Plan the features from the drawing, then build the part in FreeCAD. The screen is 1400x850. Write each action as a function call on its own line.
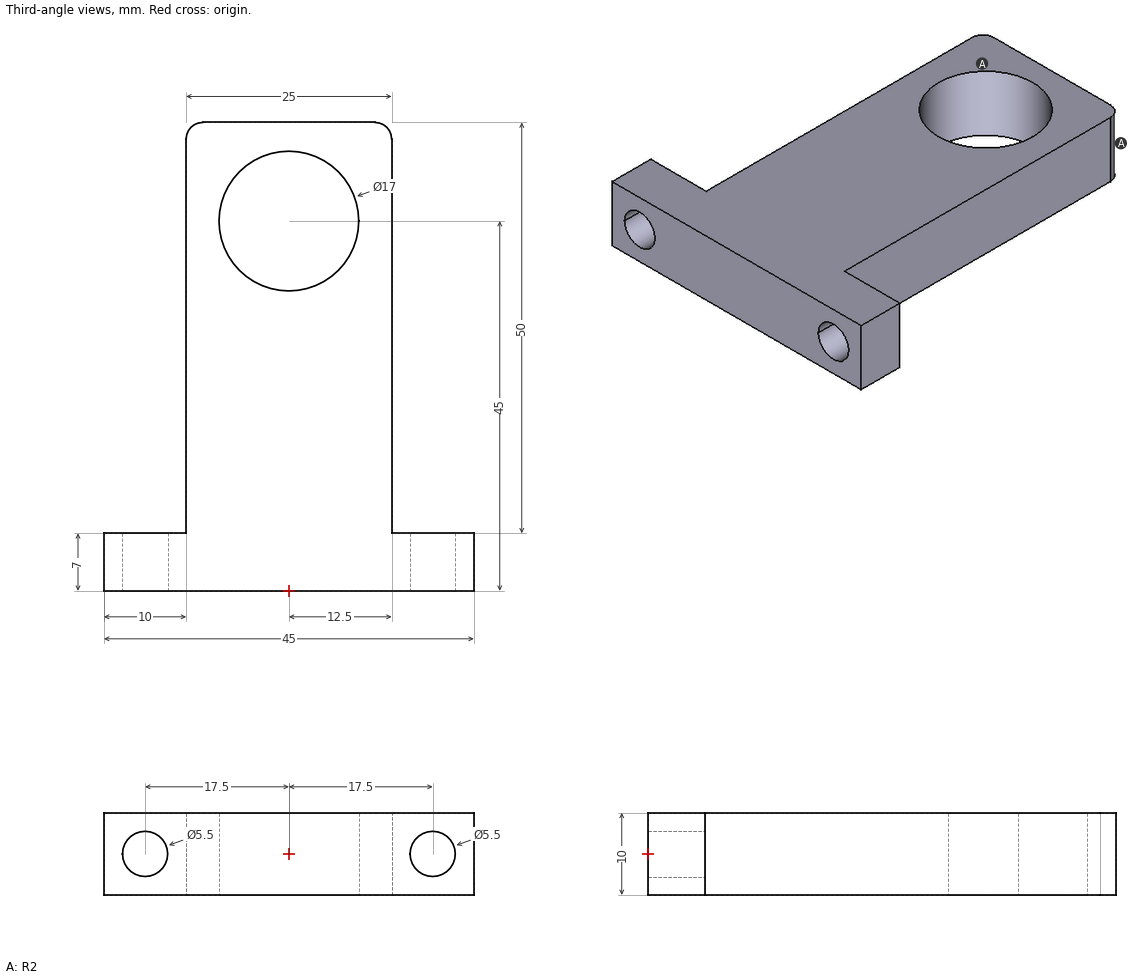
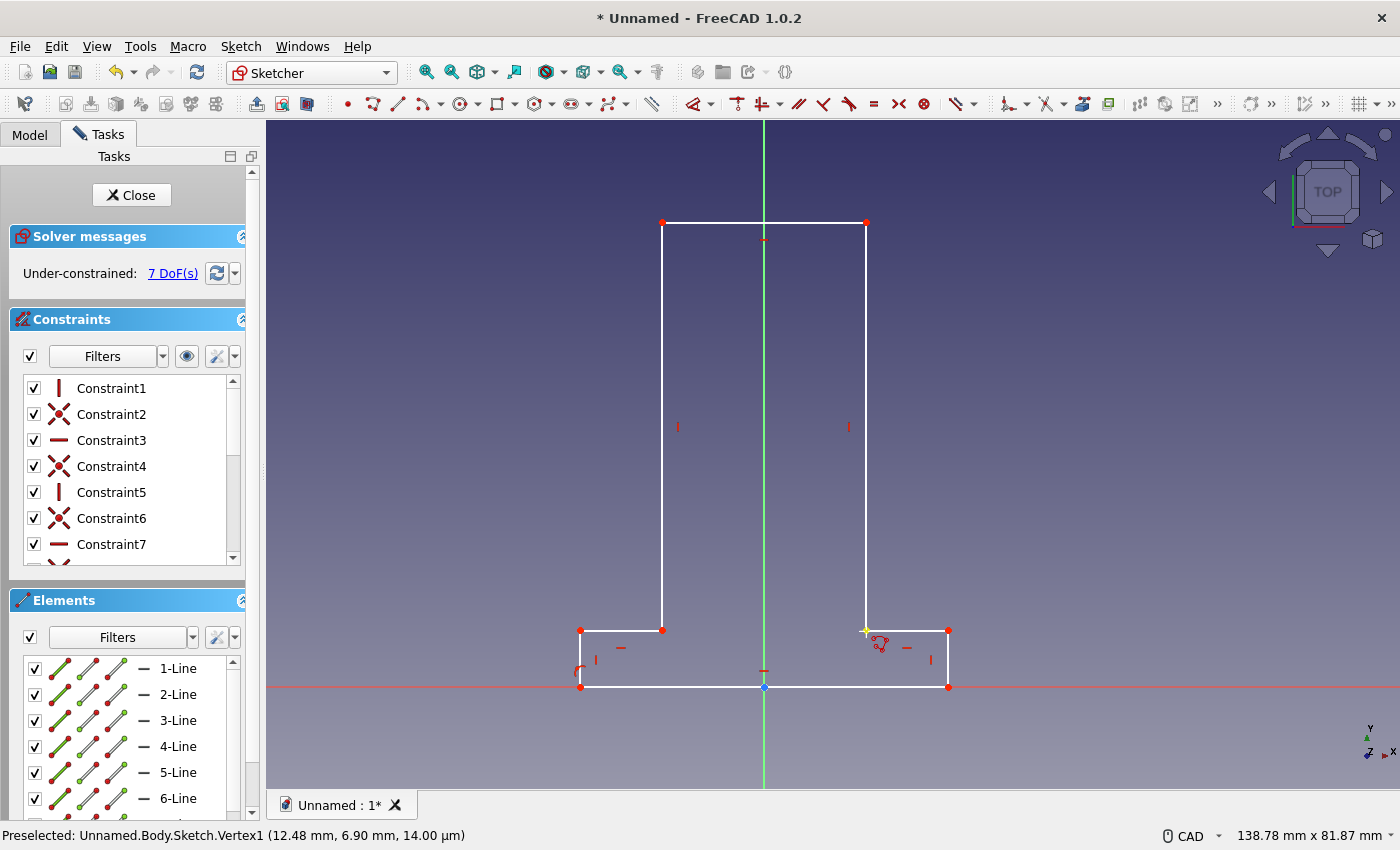
click(460, 104)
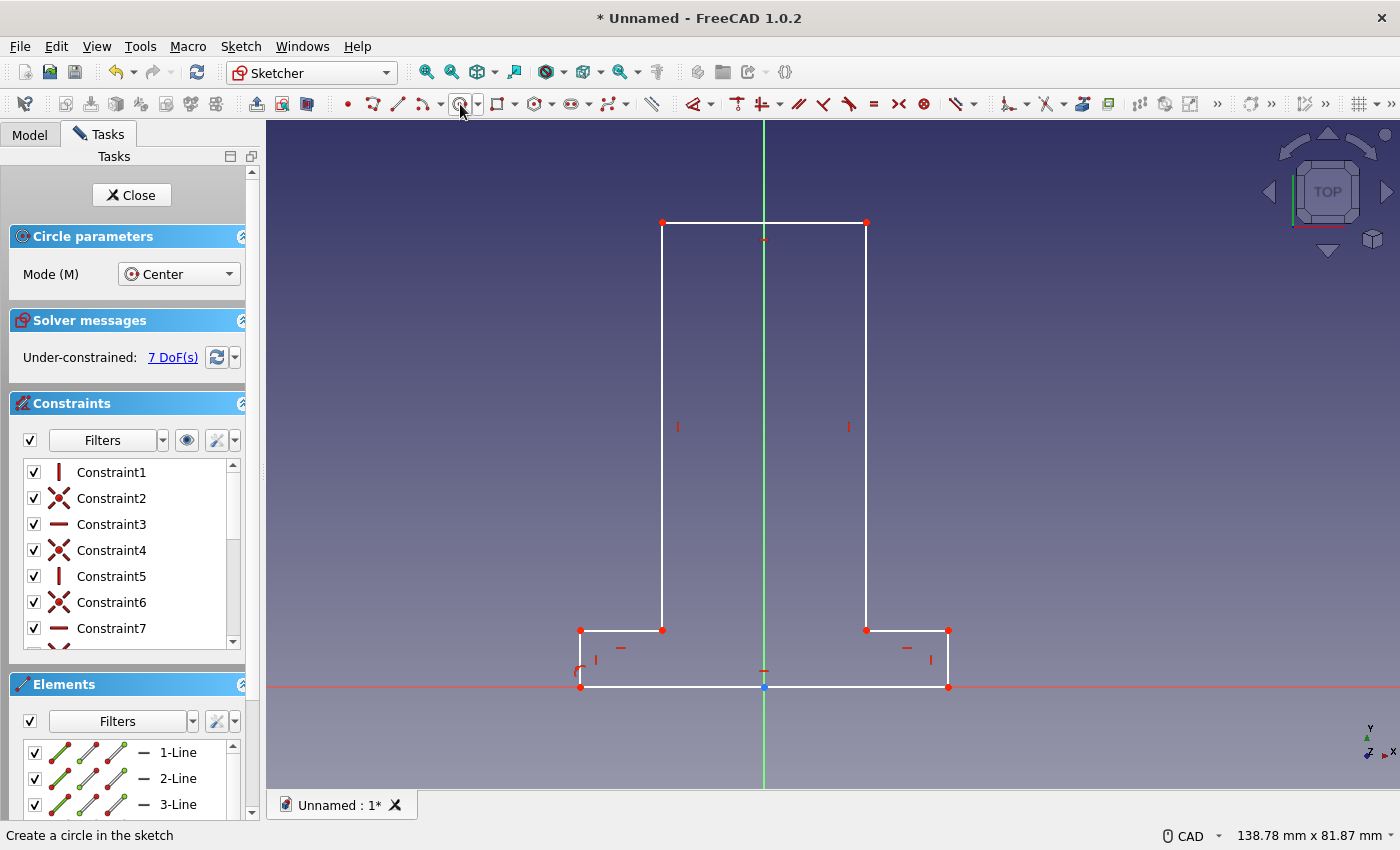
click(764, 320)
click(813, 271)
key(Escape)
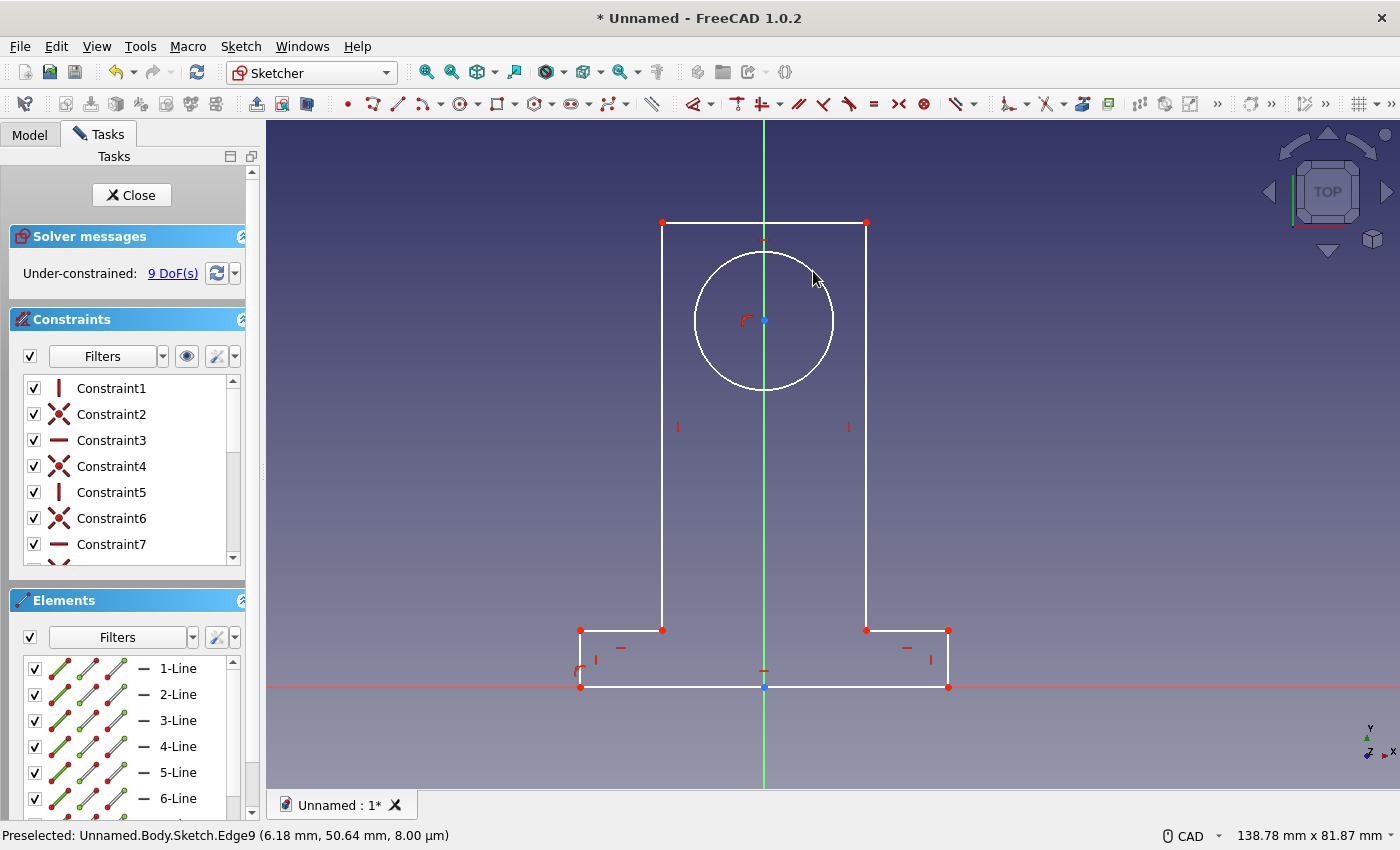
key(d)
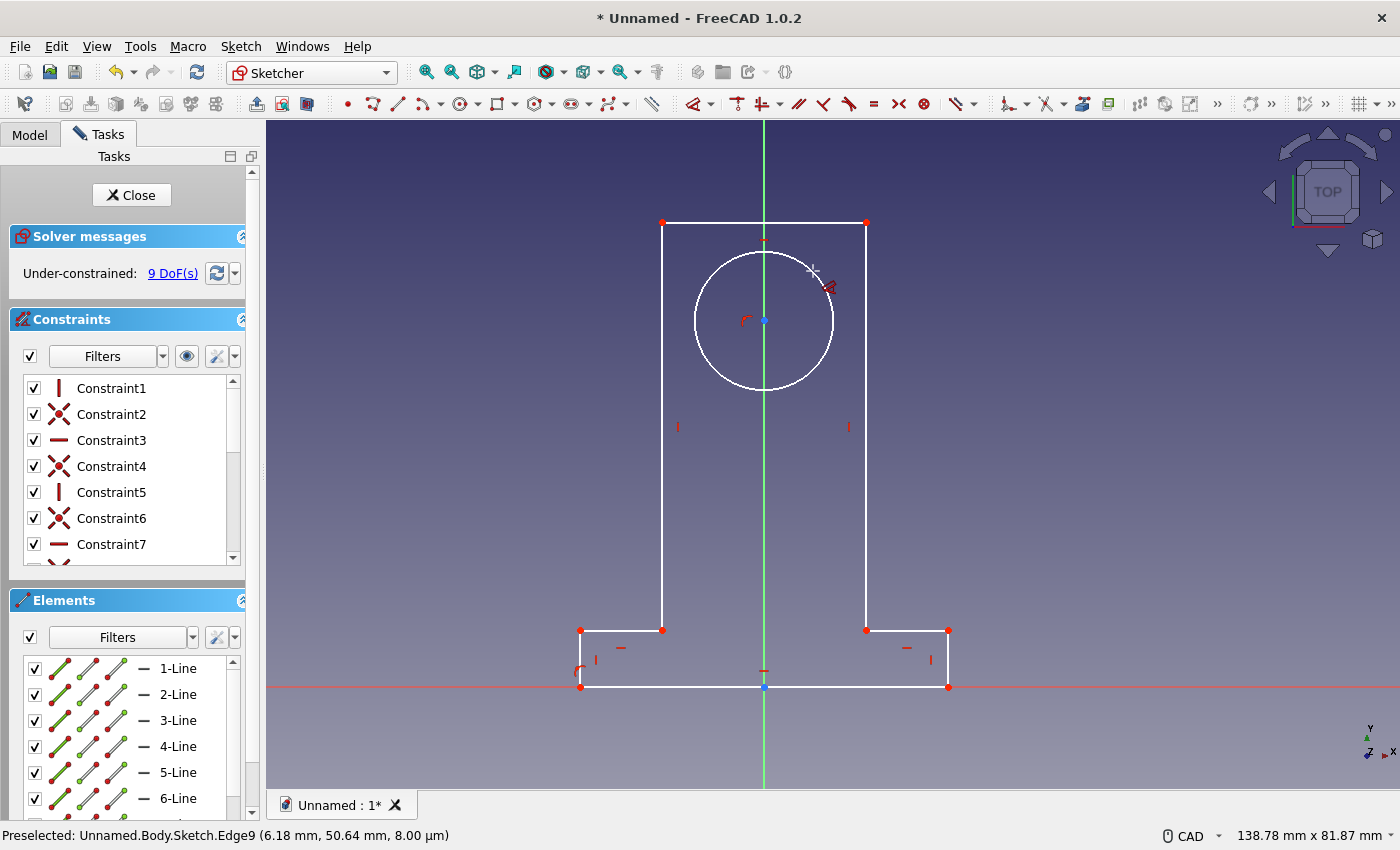
click(813, 272)
click(836, 249)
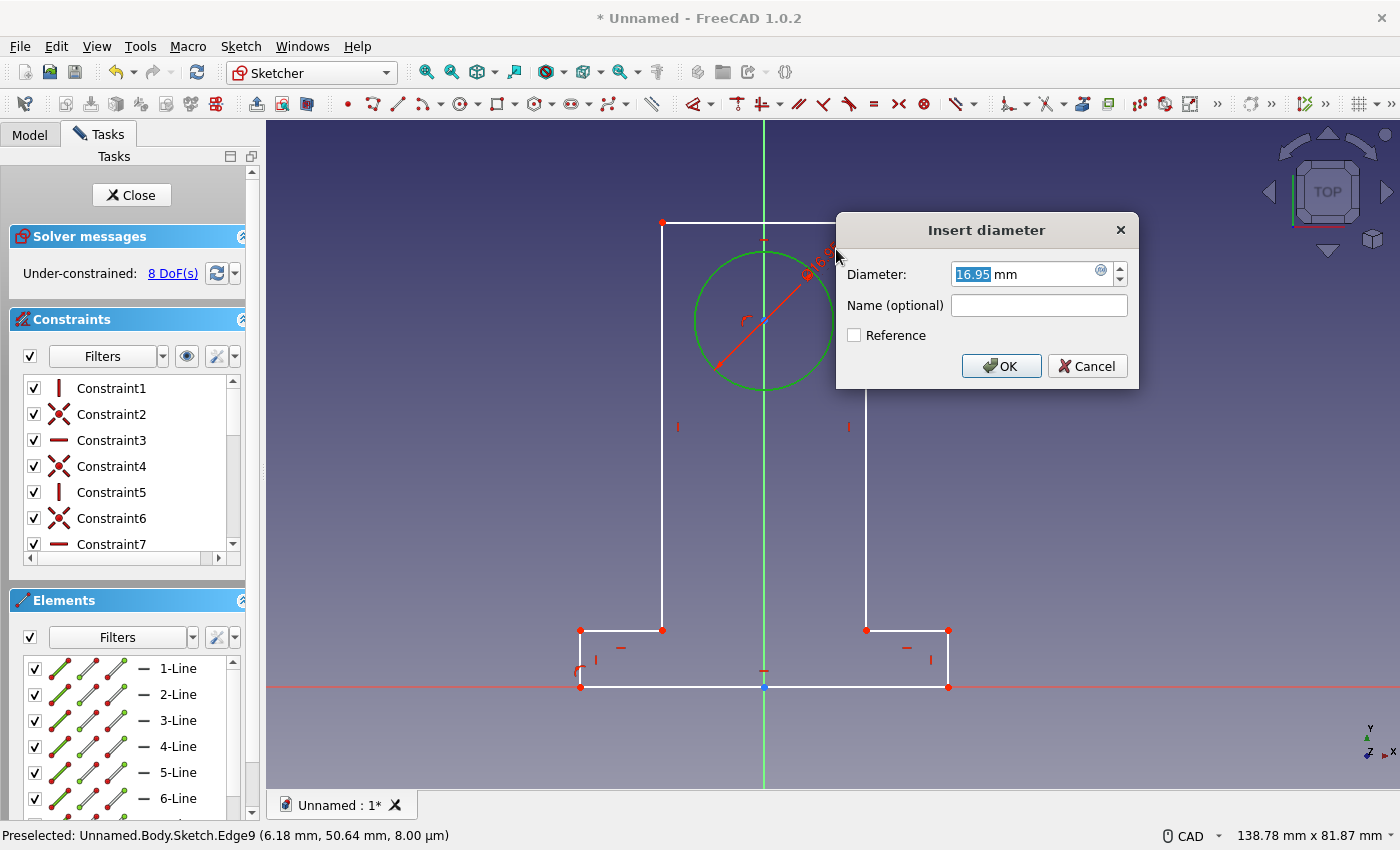
text(17)
key(Return)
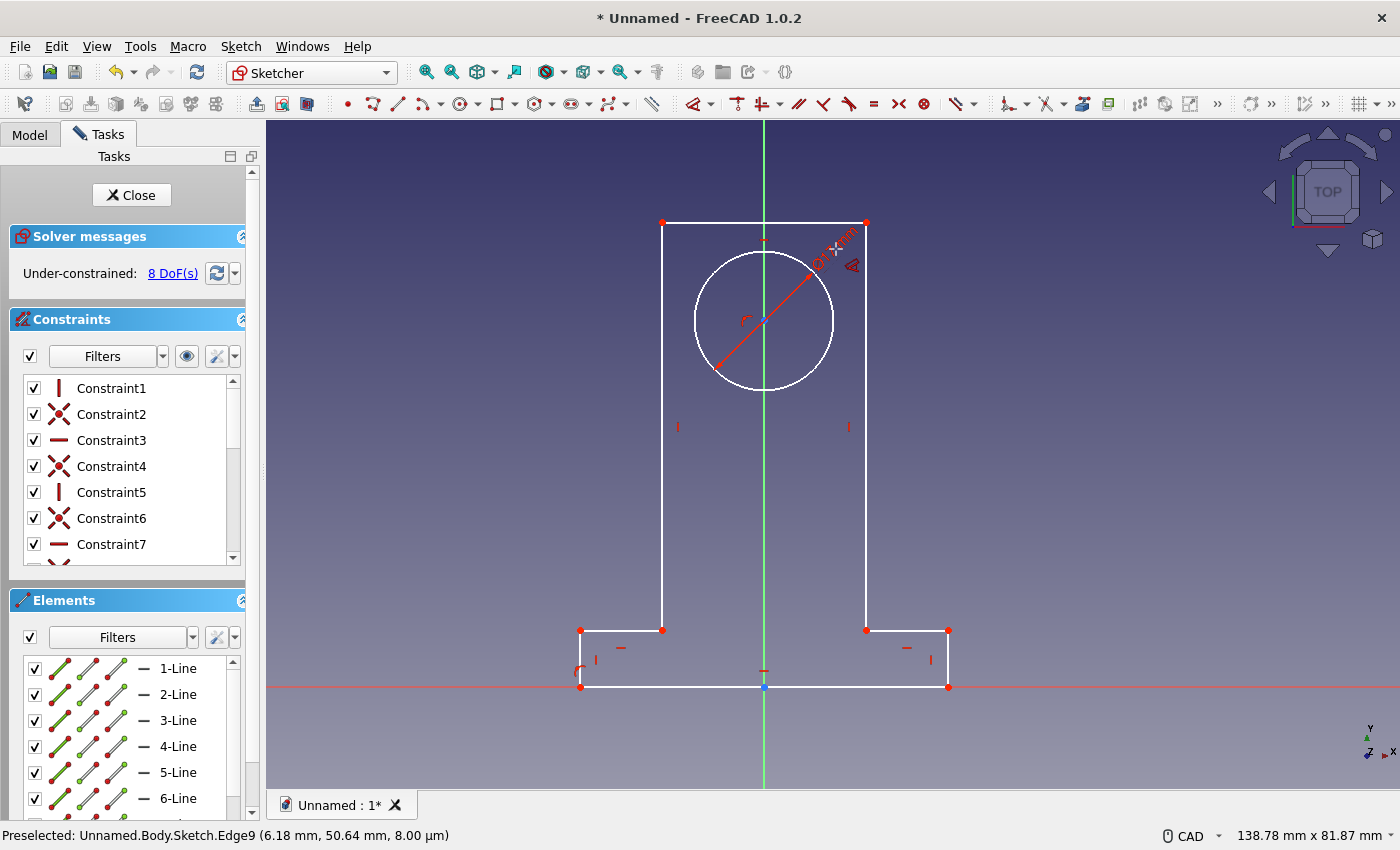
click(580, 648)
click(546, 659)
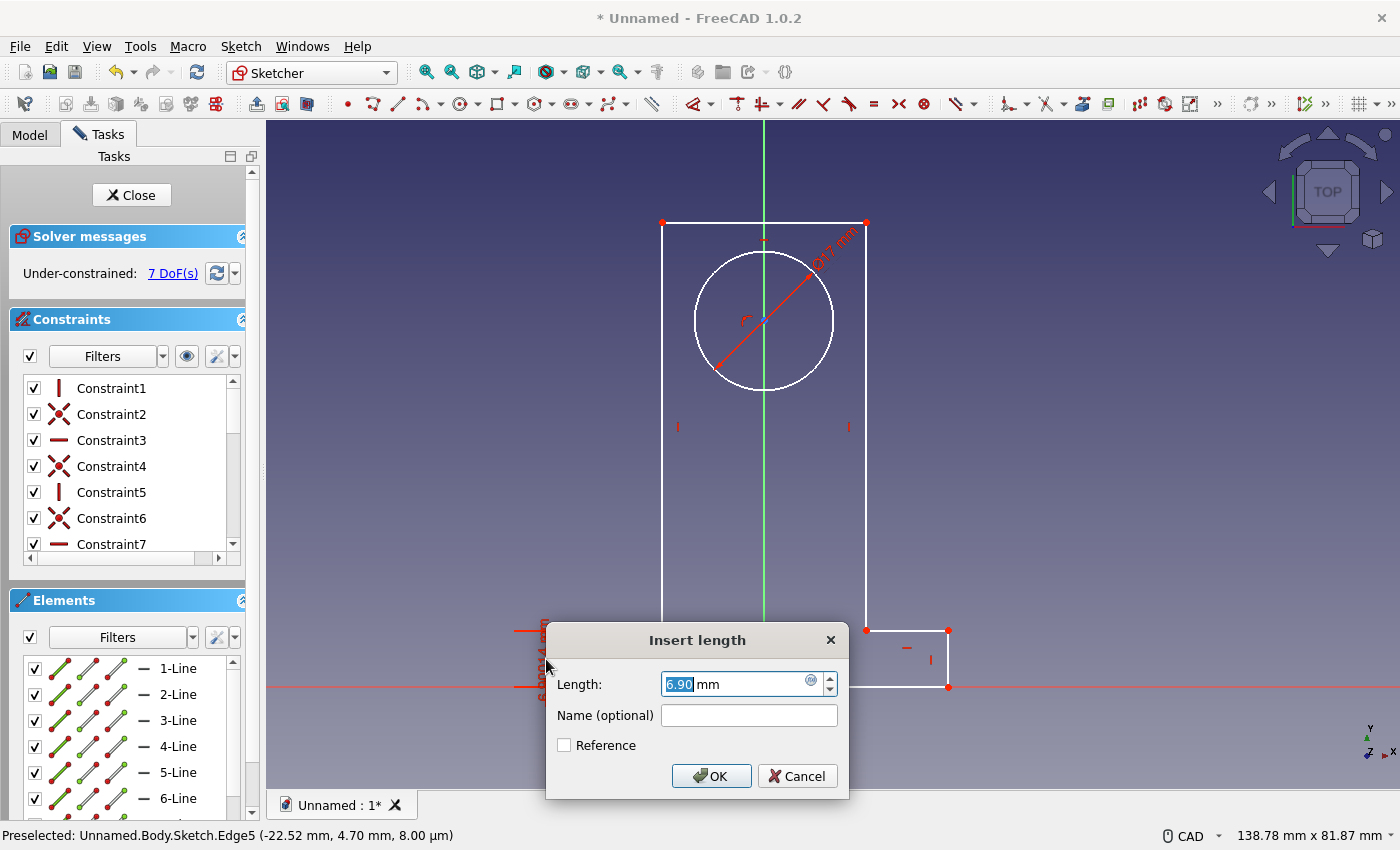
text(7)
key(Return)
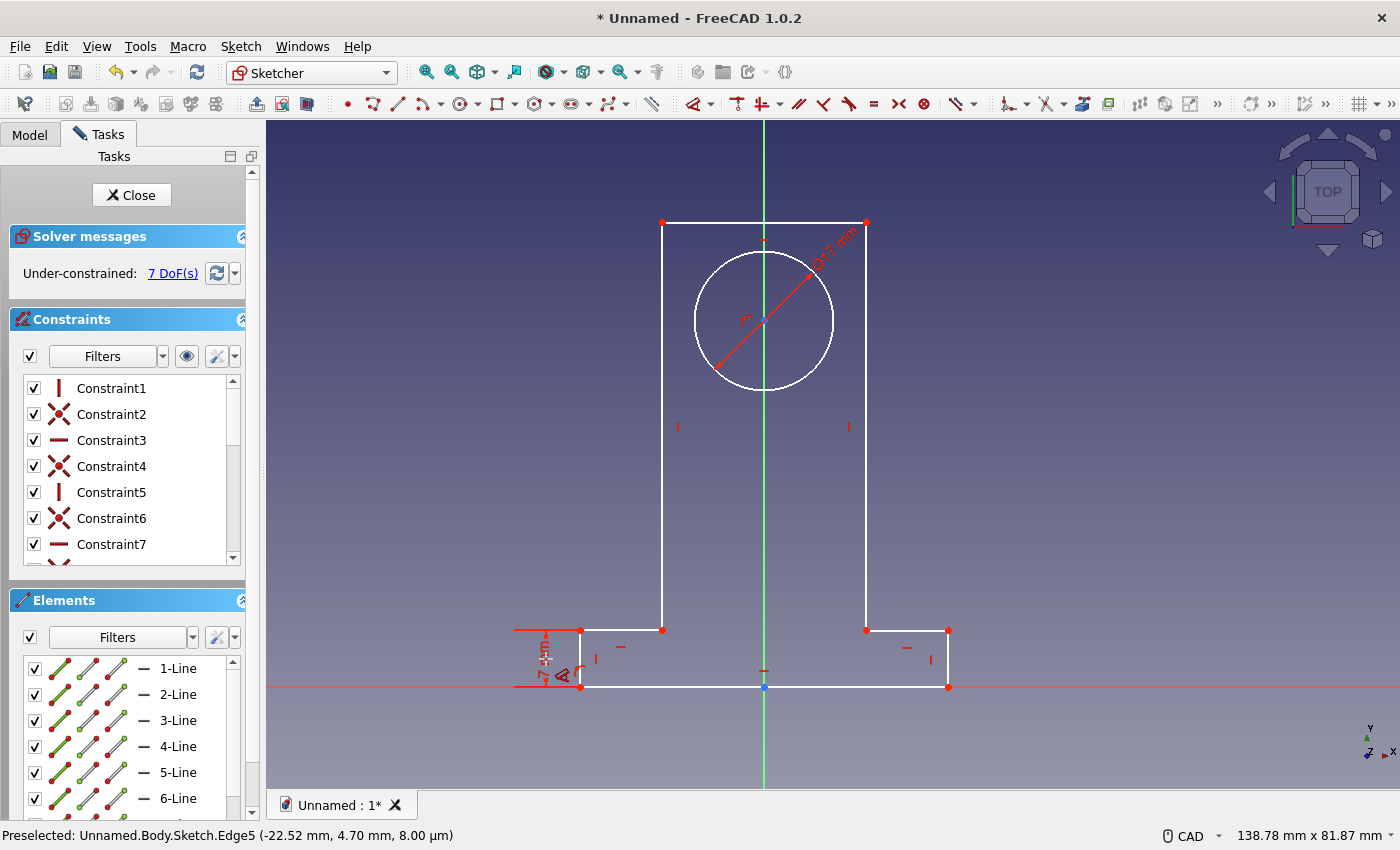
click(948, 670)
click(982, 659)